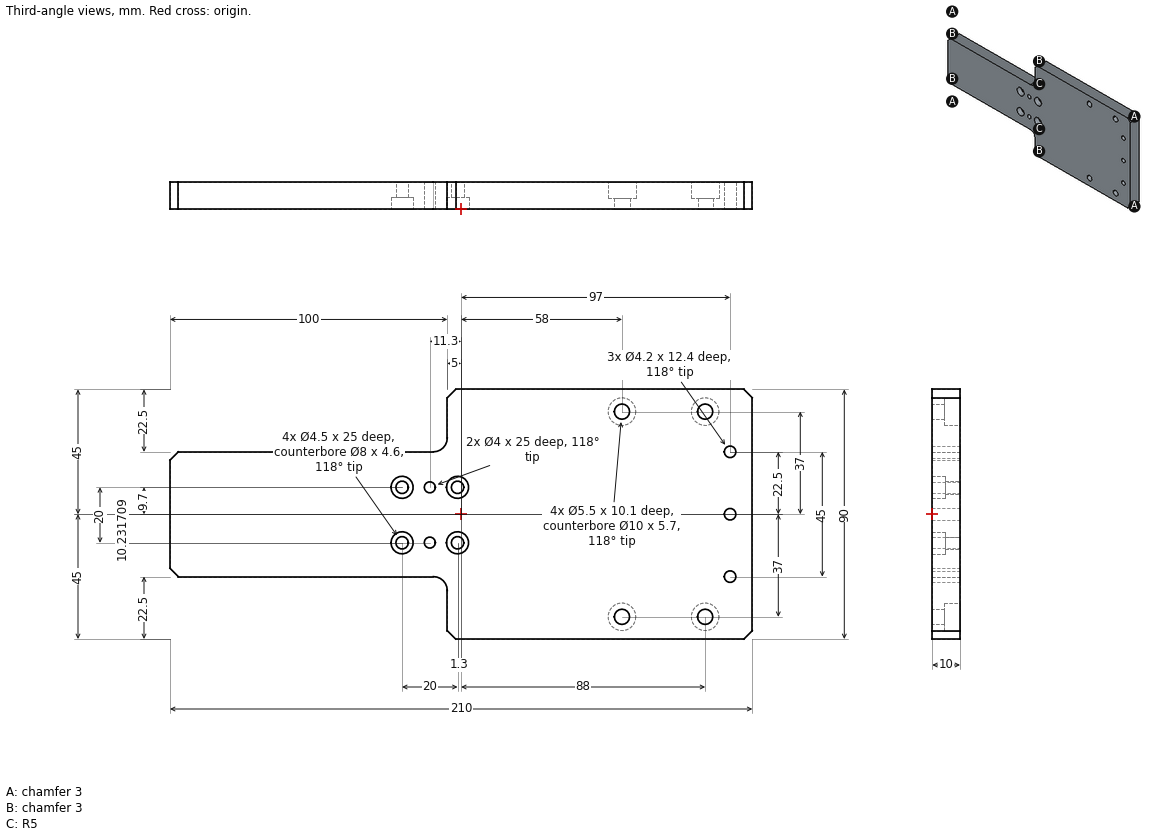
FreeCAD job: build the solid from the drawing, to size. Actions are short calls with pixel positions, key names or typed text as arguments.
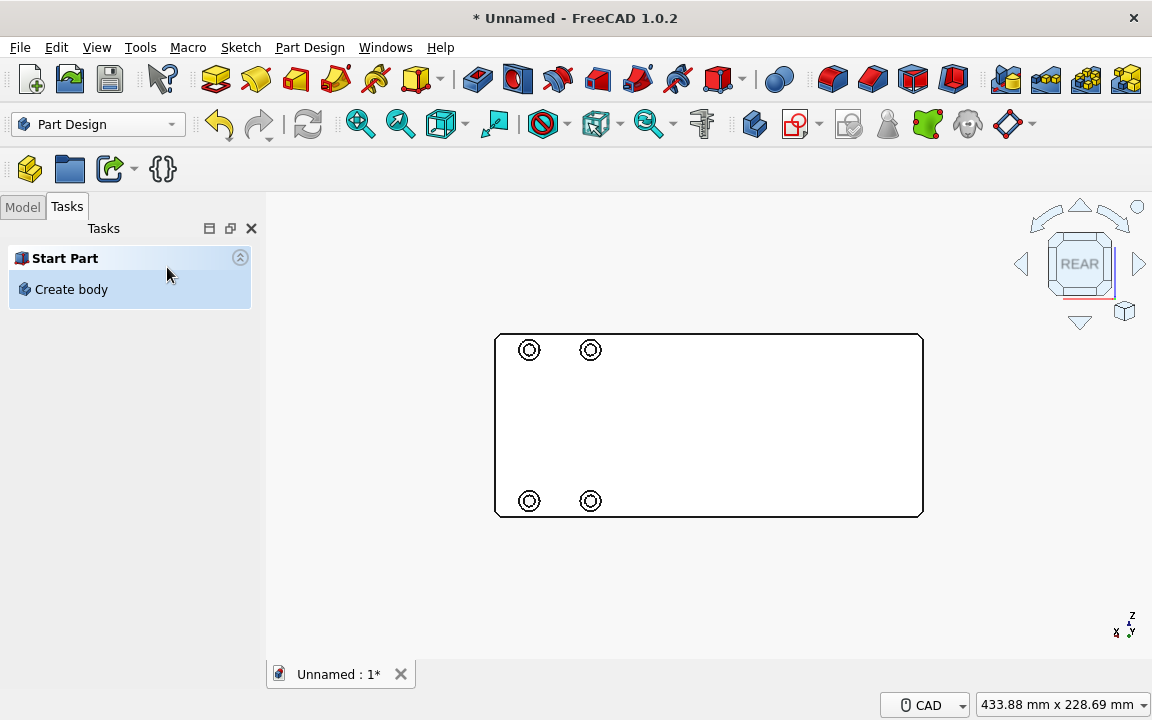
click(709, 424)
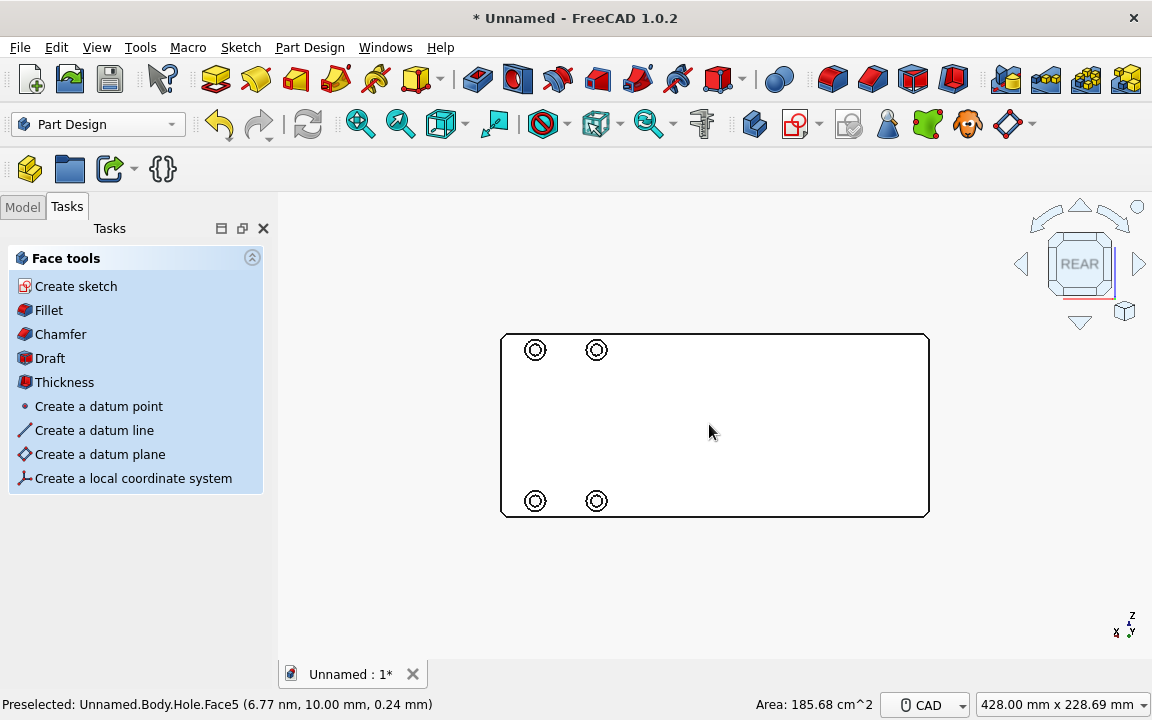
click(796, 124)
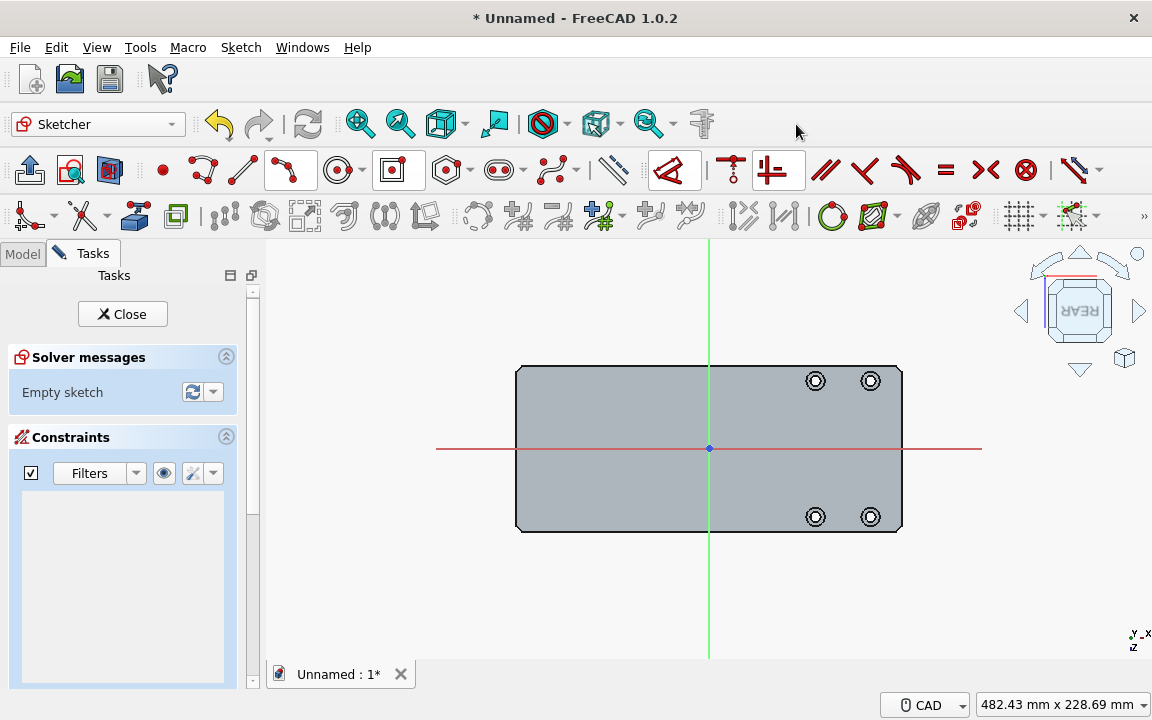
scroll(556, 449, up, 2)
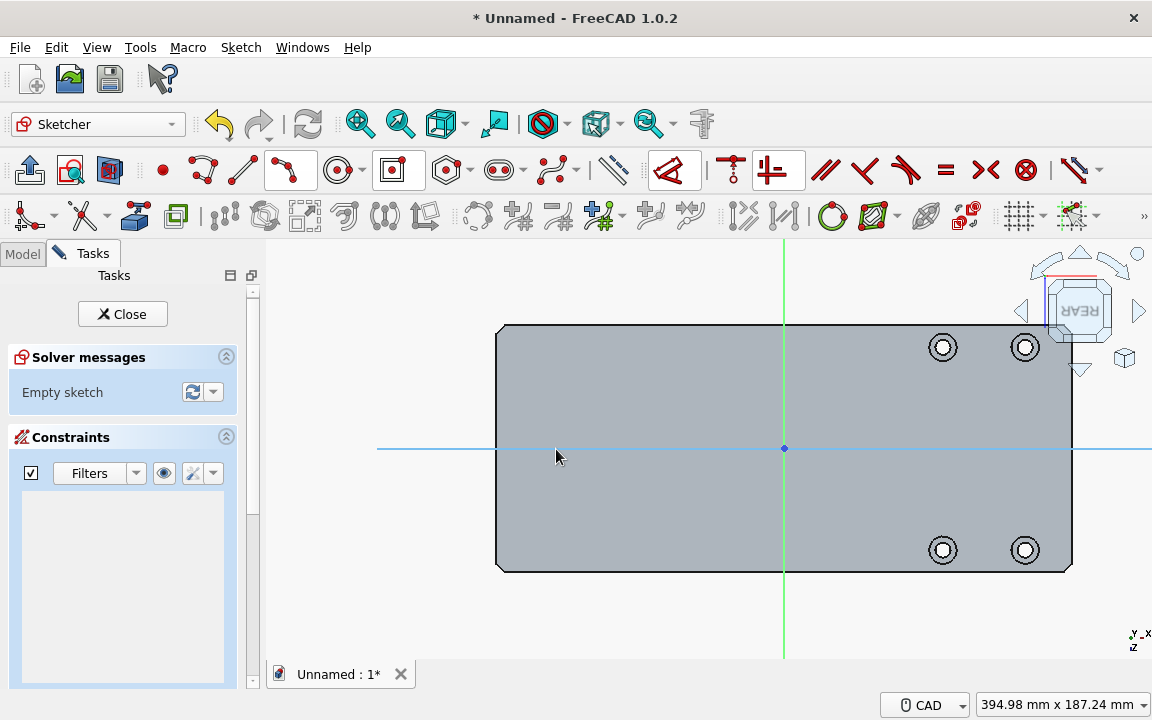
key(g)
key(r)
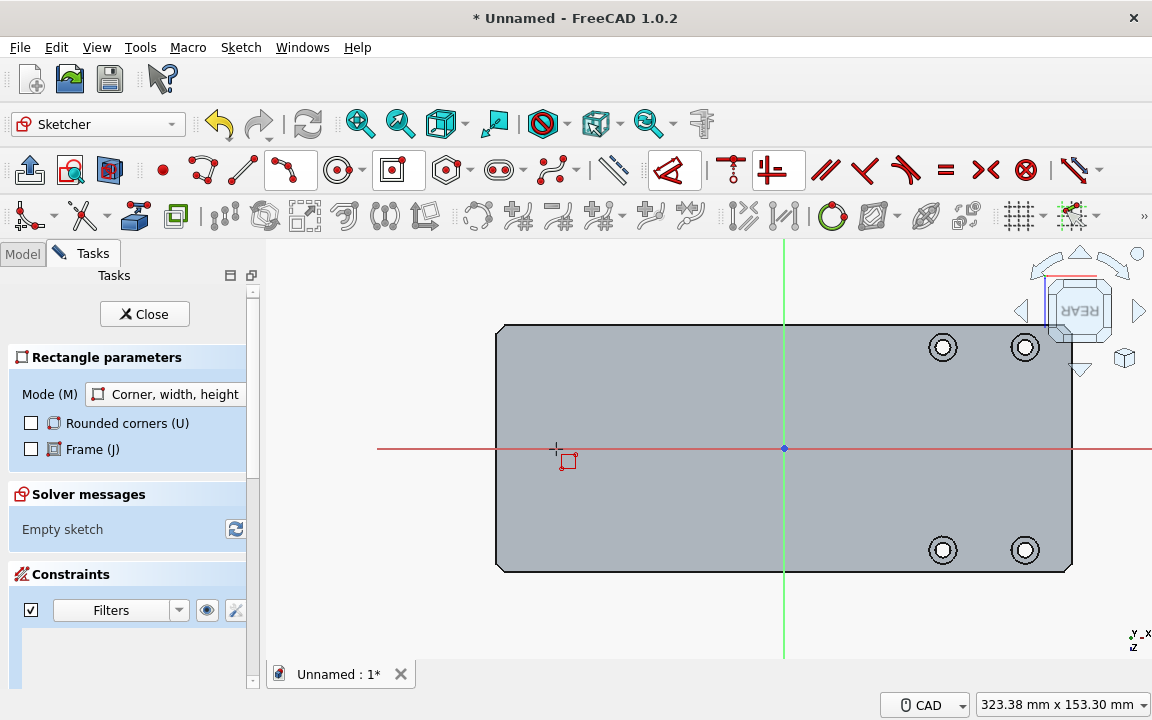
click(496, 510)
click(770, 572)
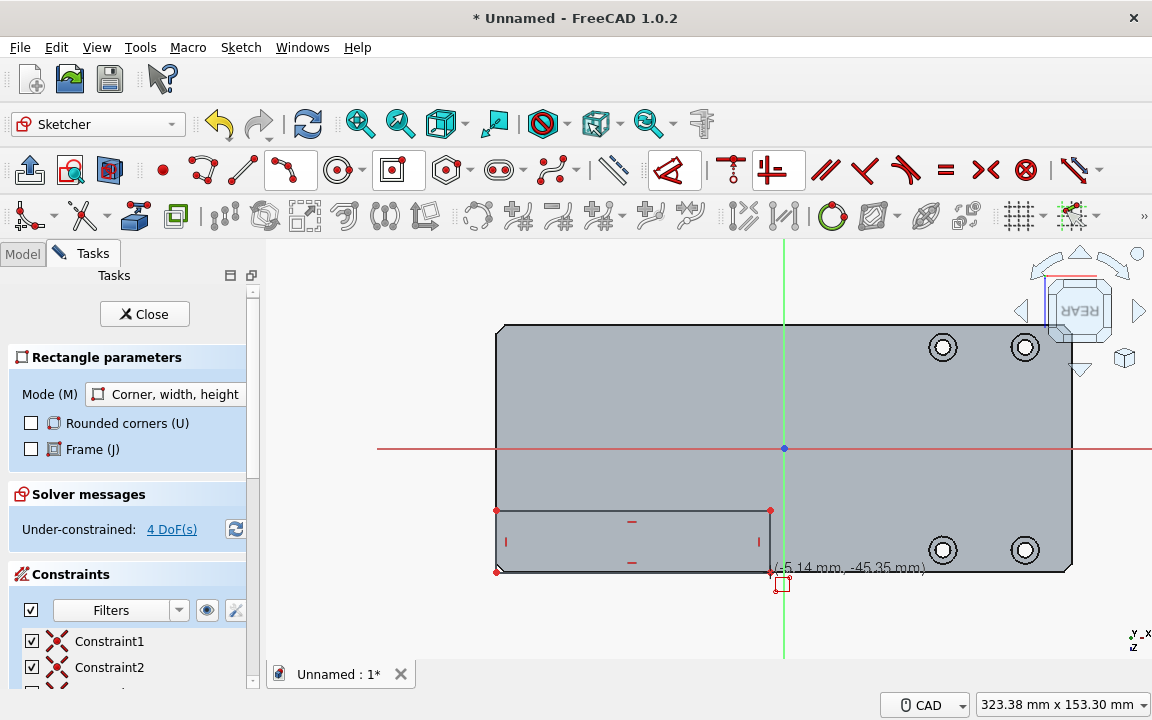
click(496, 325)
click(770, 387)
key(Escape)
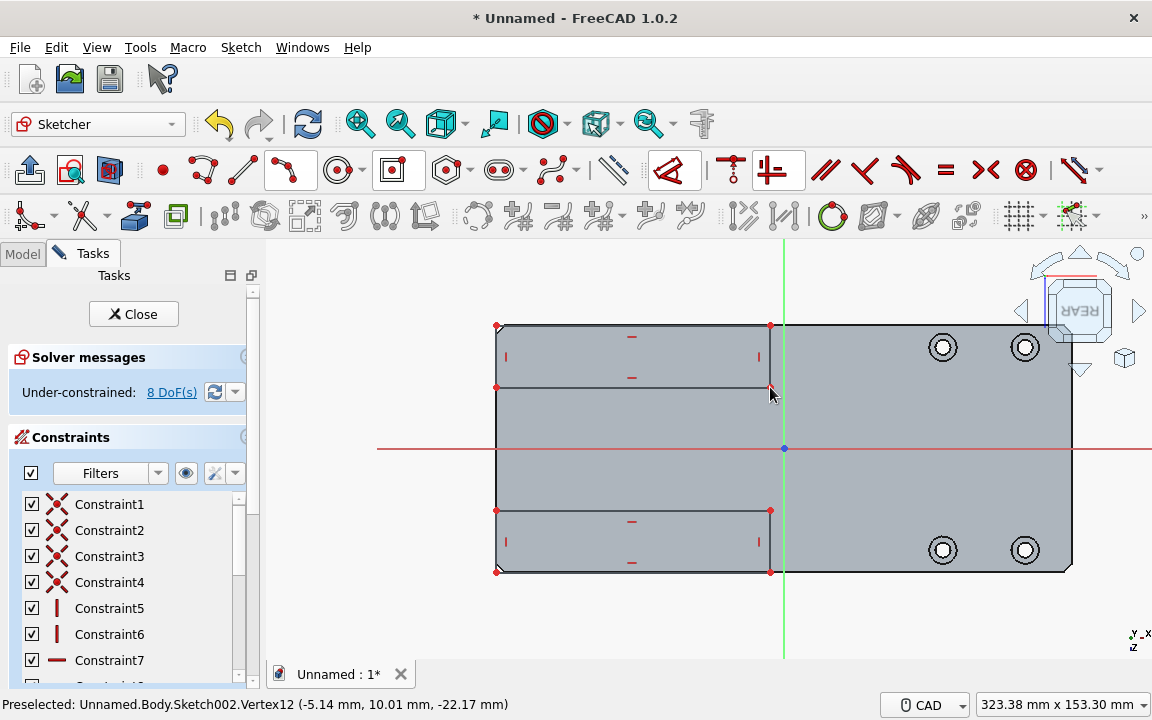
scroll(770, 573, up, 6)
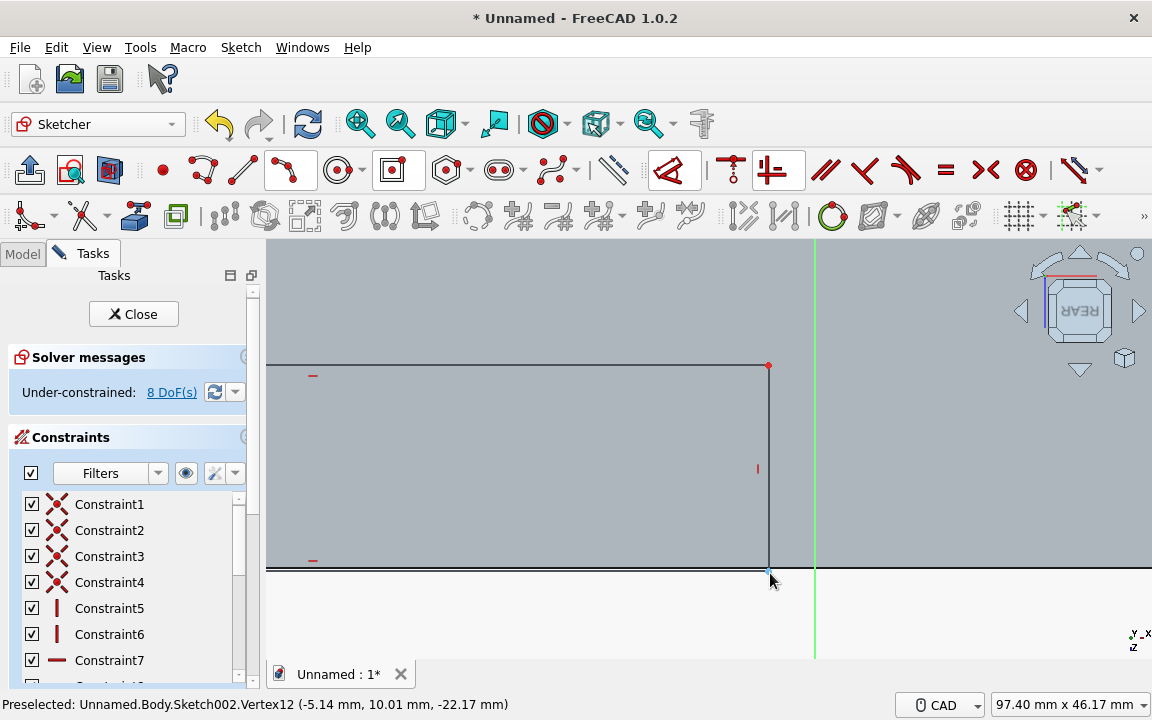
click(769, 571)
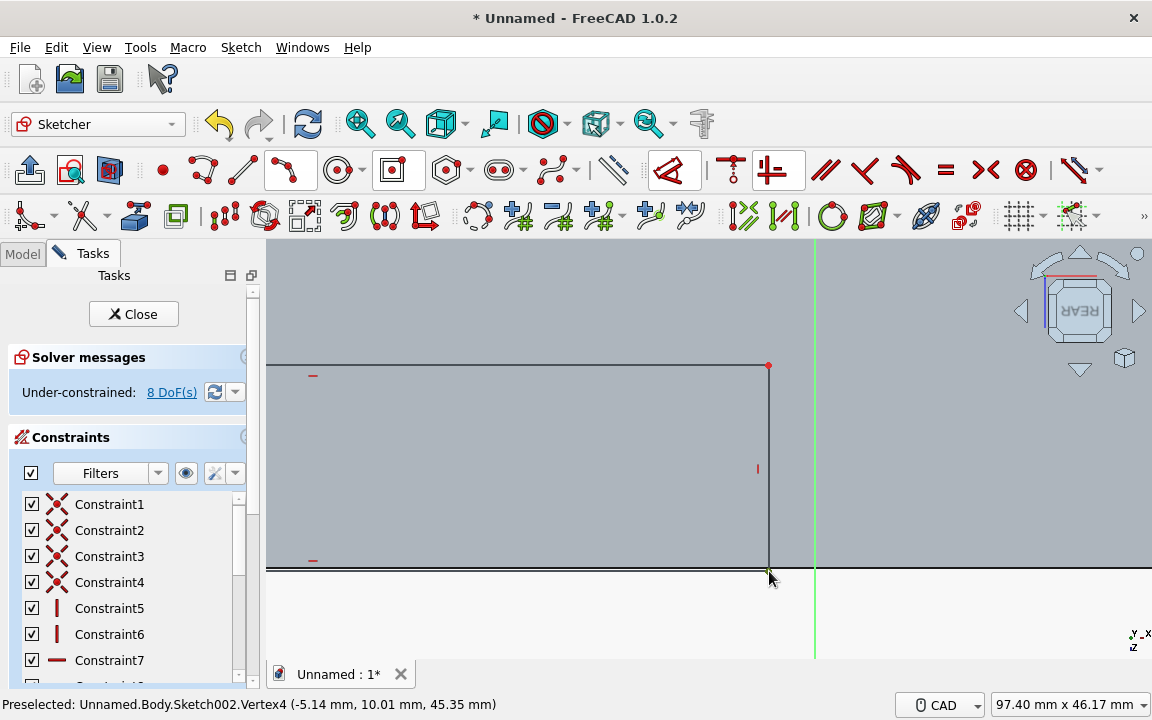
click(696, 170)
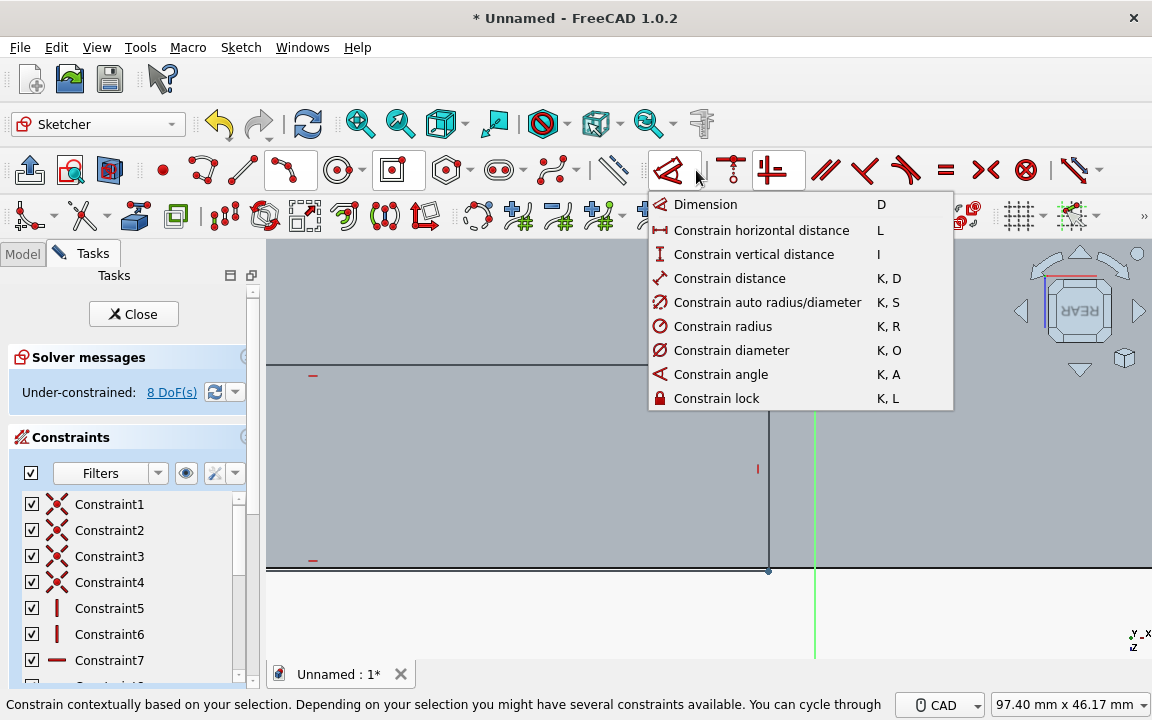
click(801, 230)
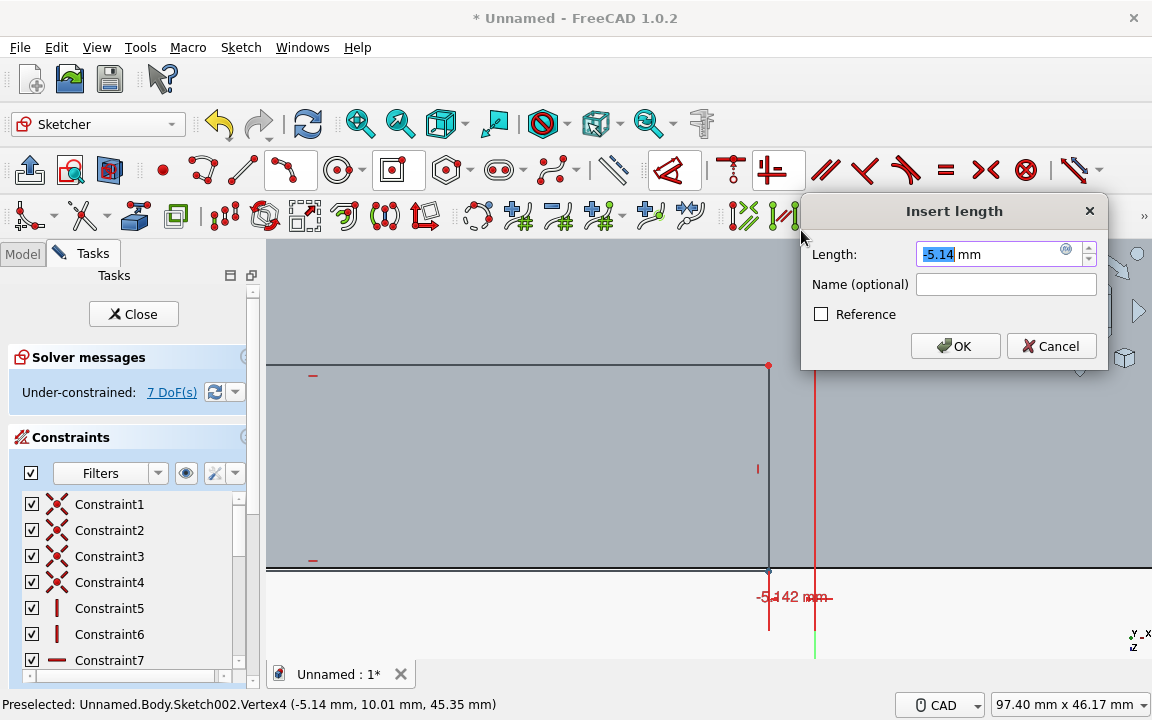
text(-5)
key(Return)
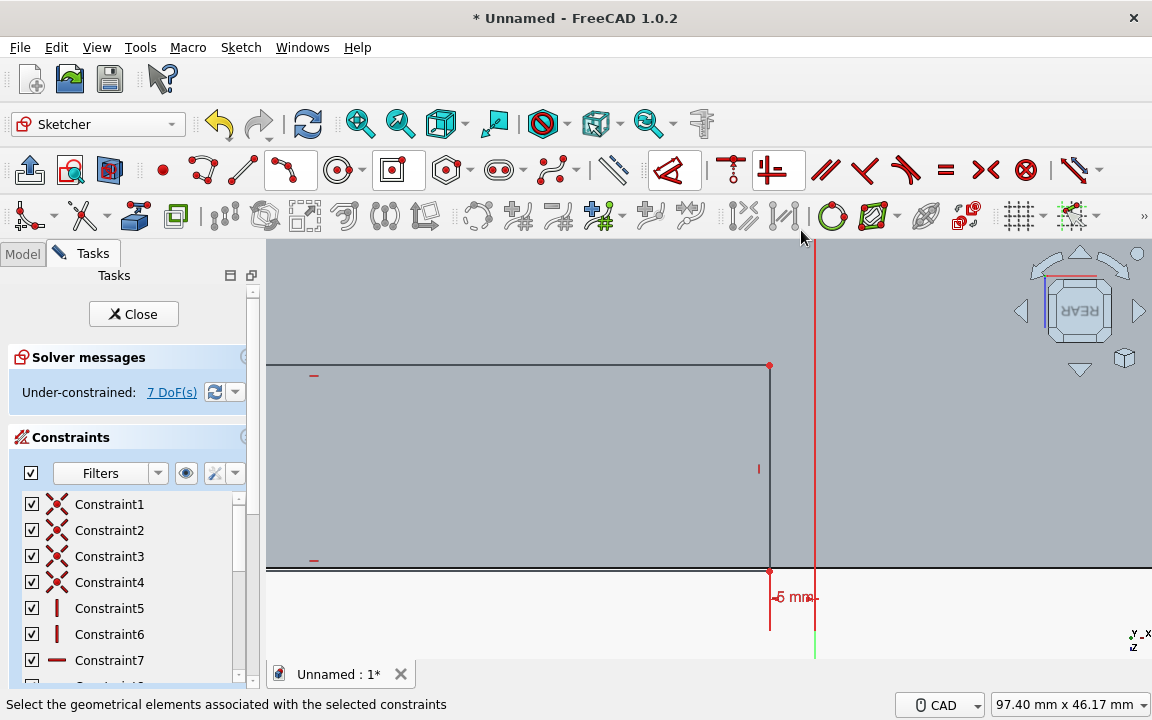
scroll(771, 574, down, 6)